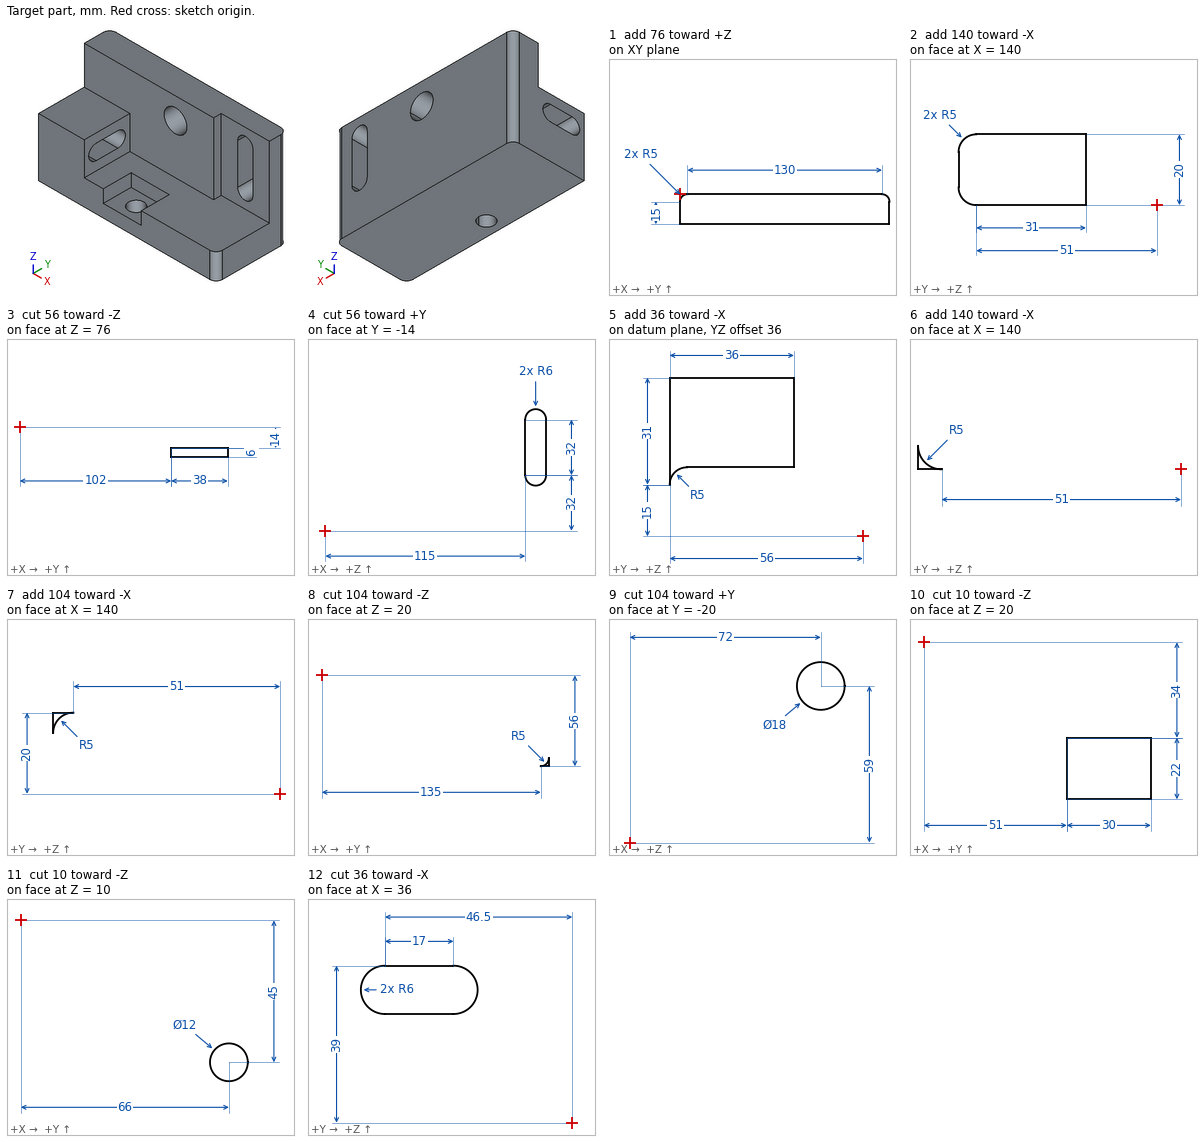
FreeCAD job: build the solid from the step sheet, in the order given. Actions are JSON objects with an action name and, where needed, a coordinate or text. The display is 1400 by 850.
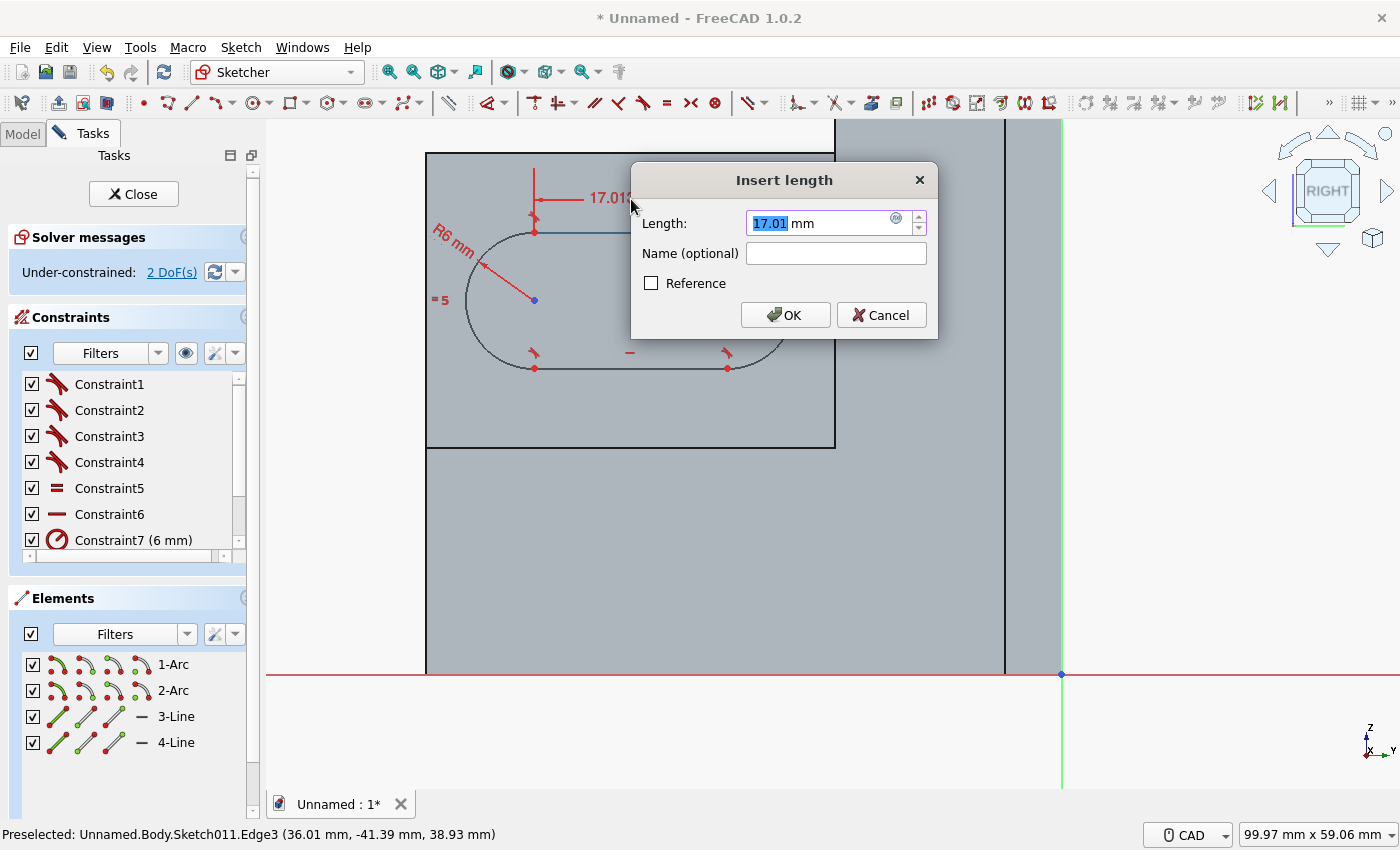
{"action": "type", "text": "17"}
{"action": "key", "text": "Return"}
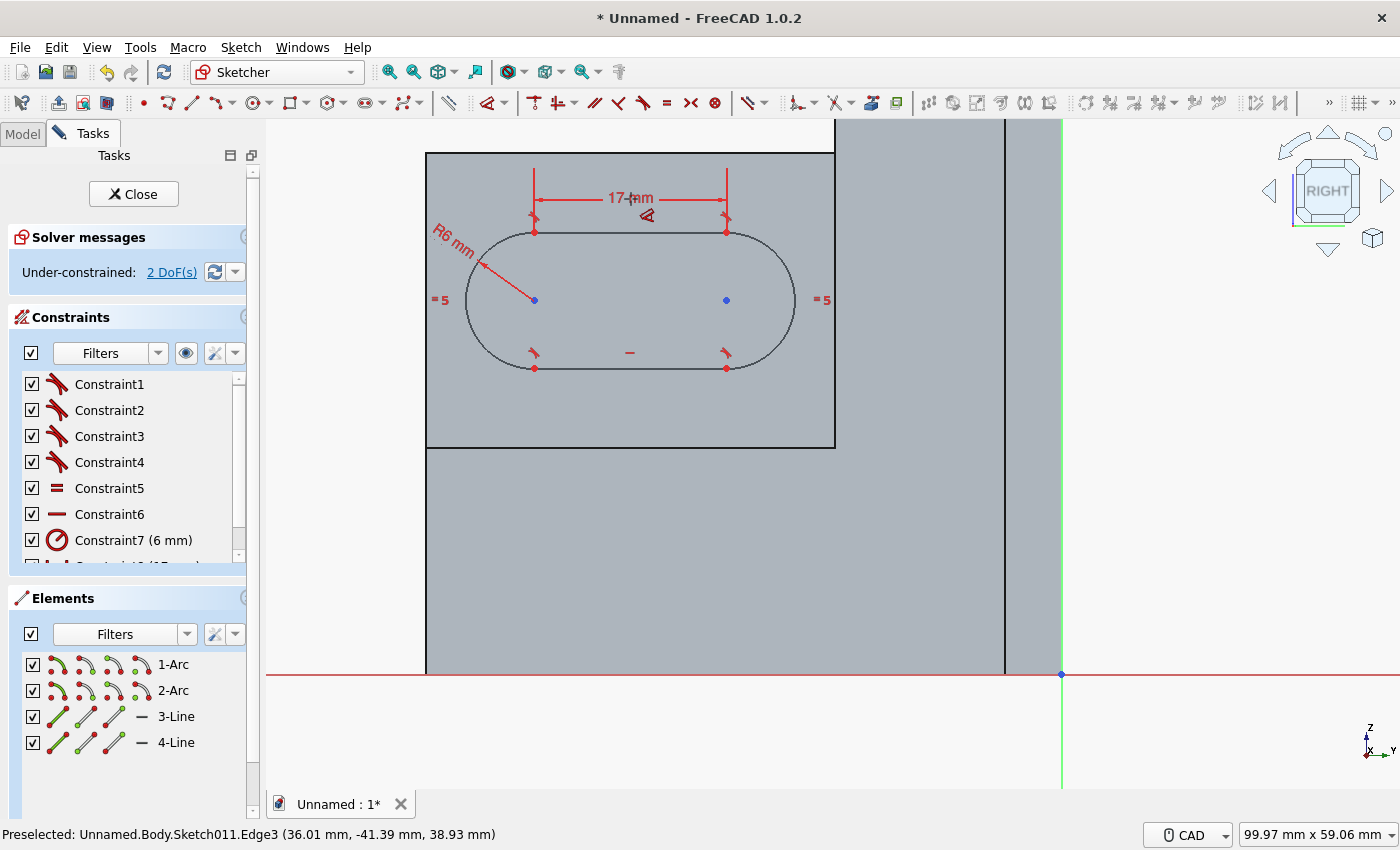
{"action": "left_click", "coordinate": [534, 233]}
{"action": "left_click", "coordinate": [1096, 454]}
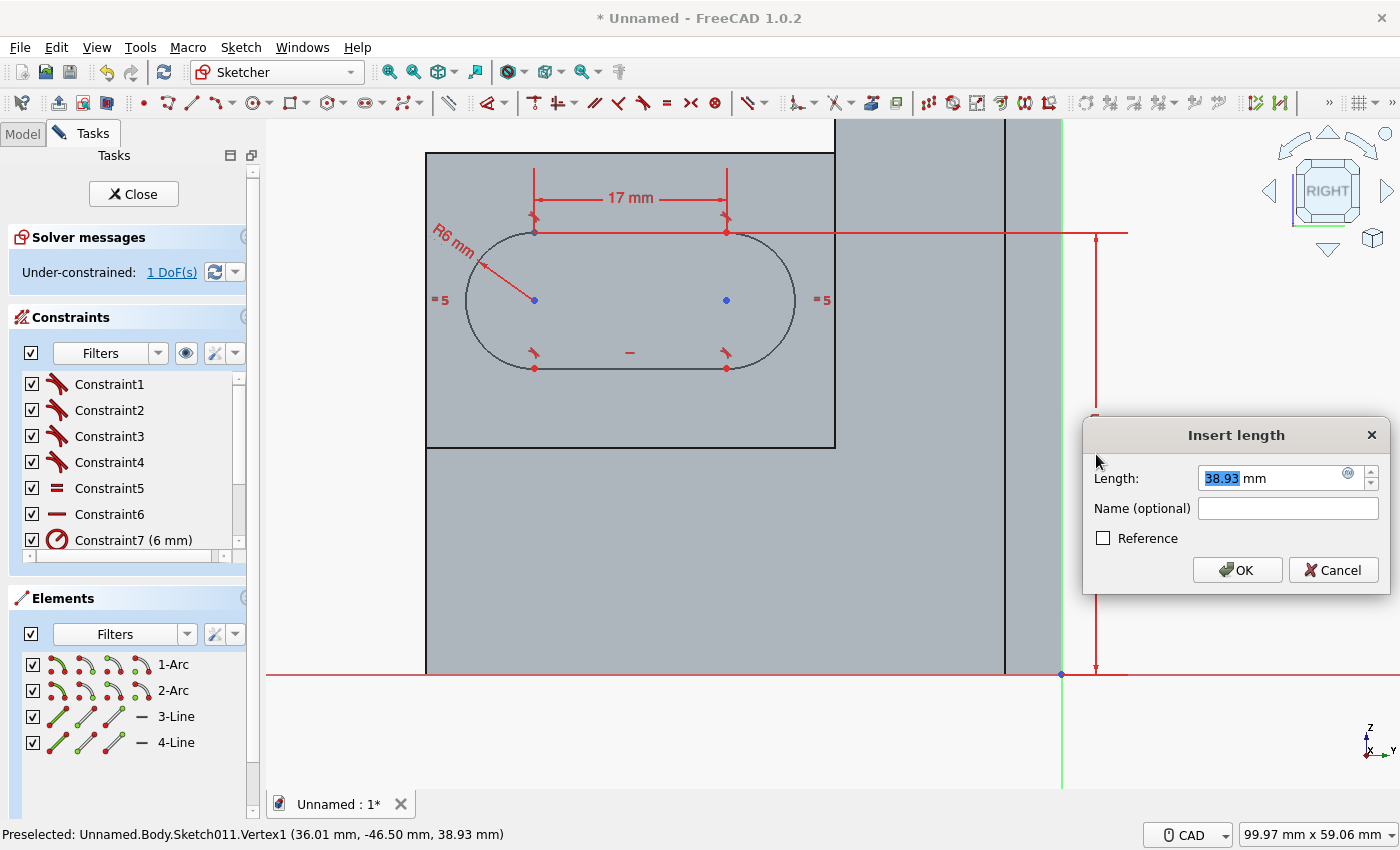
{"action": "type", "text": "39"}
{"action": "key", "text": "Return"}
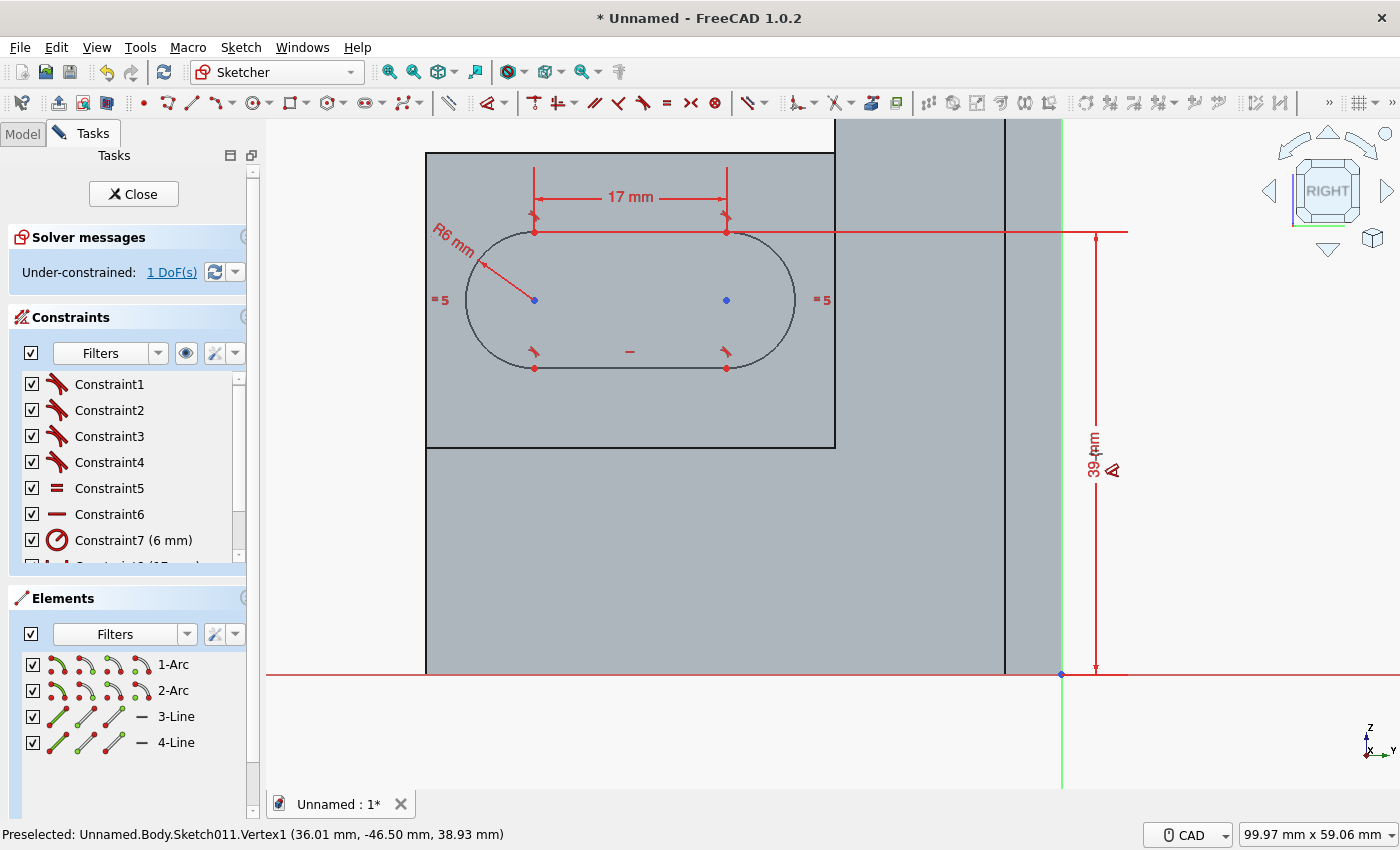
{"action": "left_click", "coordinate": [534, 232]}
{"action": "left_click", "coordinate": [798, 709]}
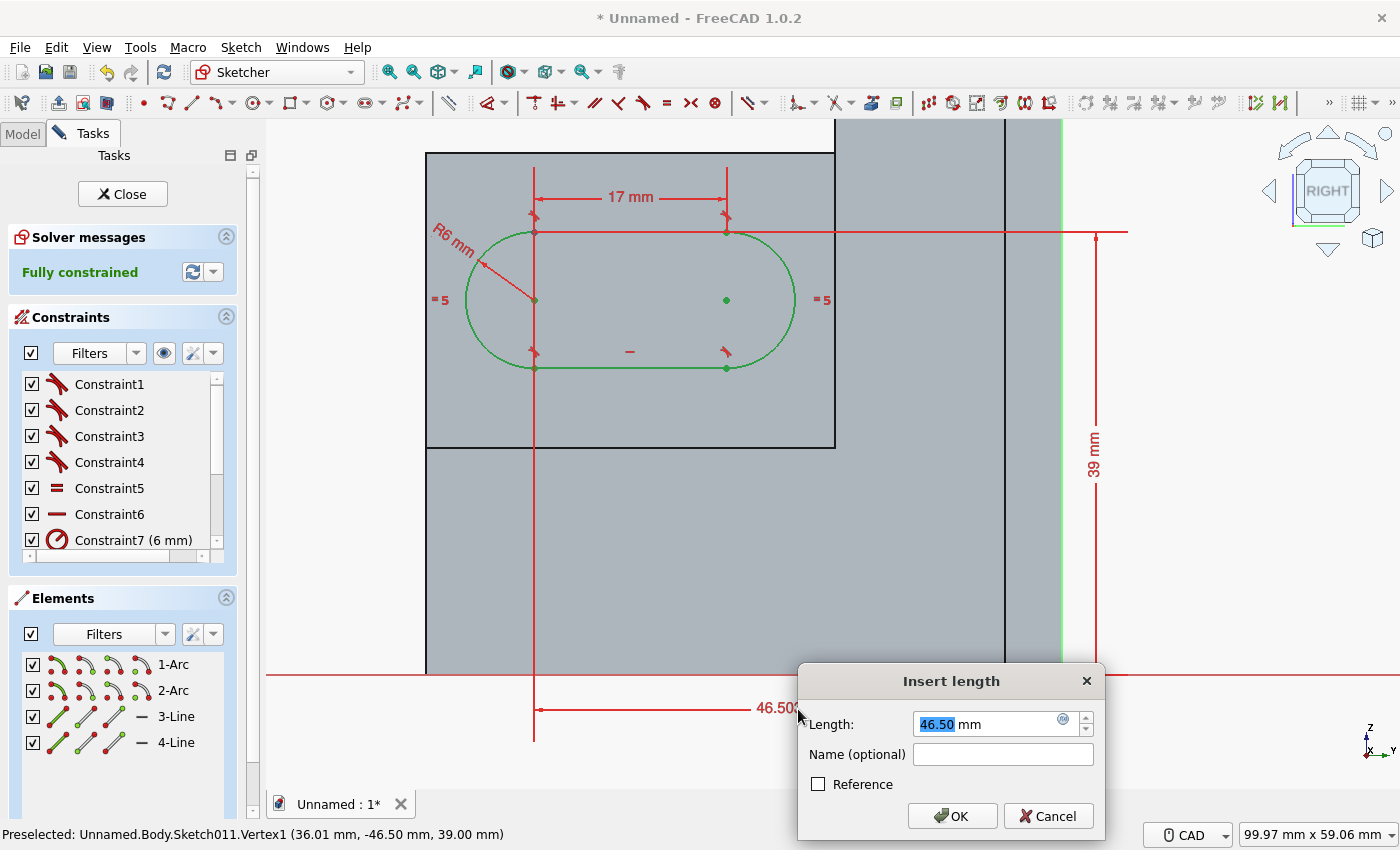
{"action": "type", "text": "46.5"}
{"action": "key", "text": "Return"}
{"action": "key", "text": "Escape"}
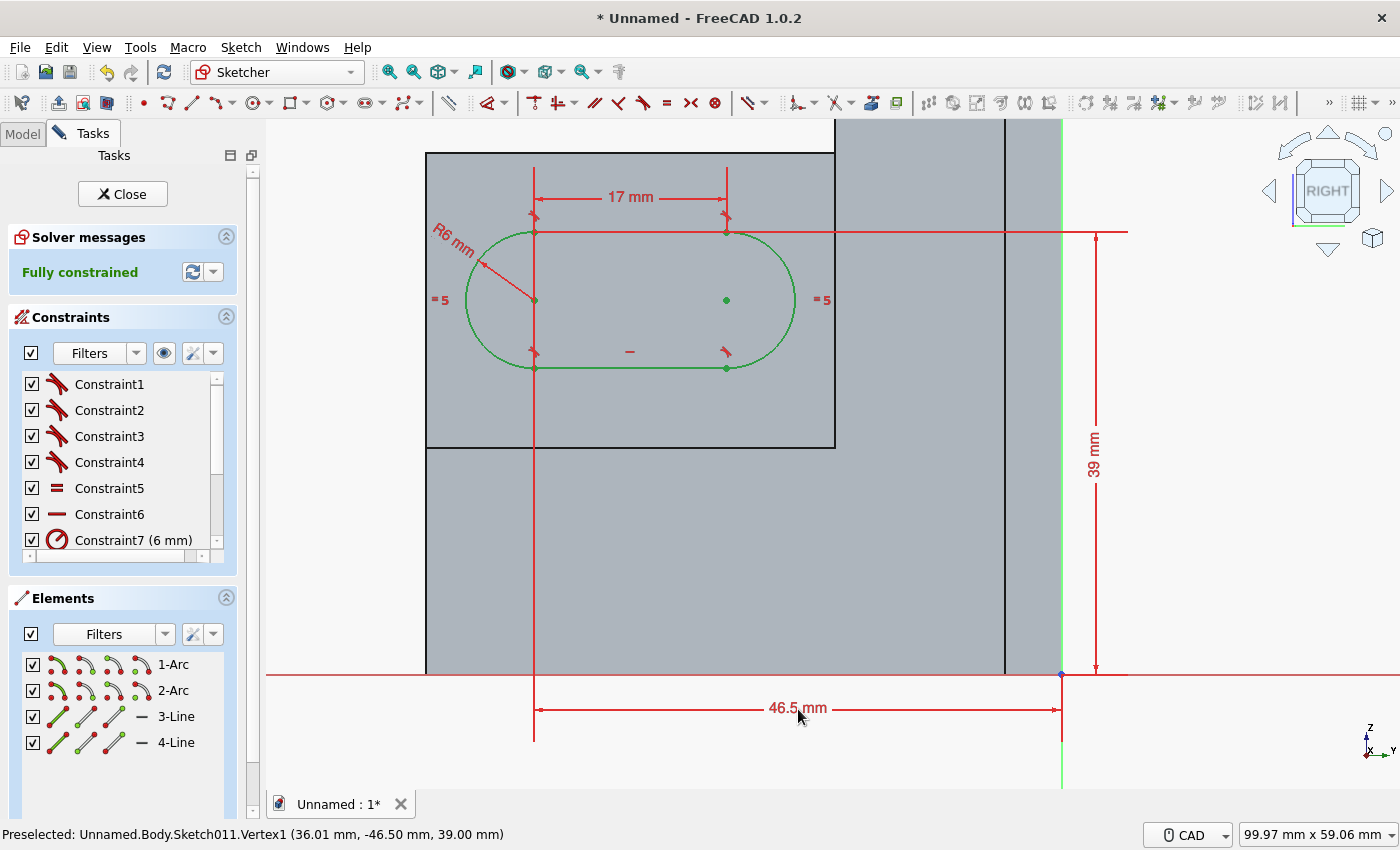
{"action": "left_click", "coordinate": [123, 194]}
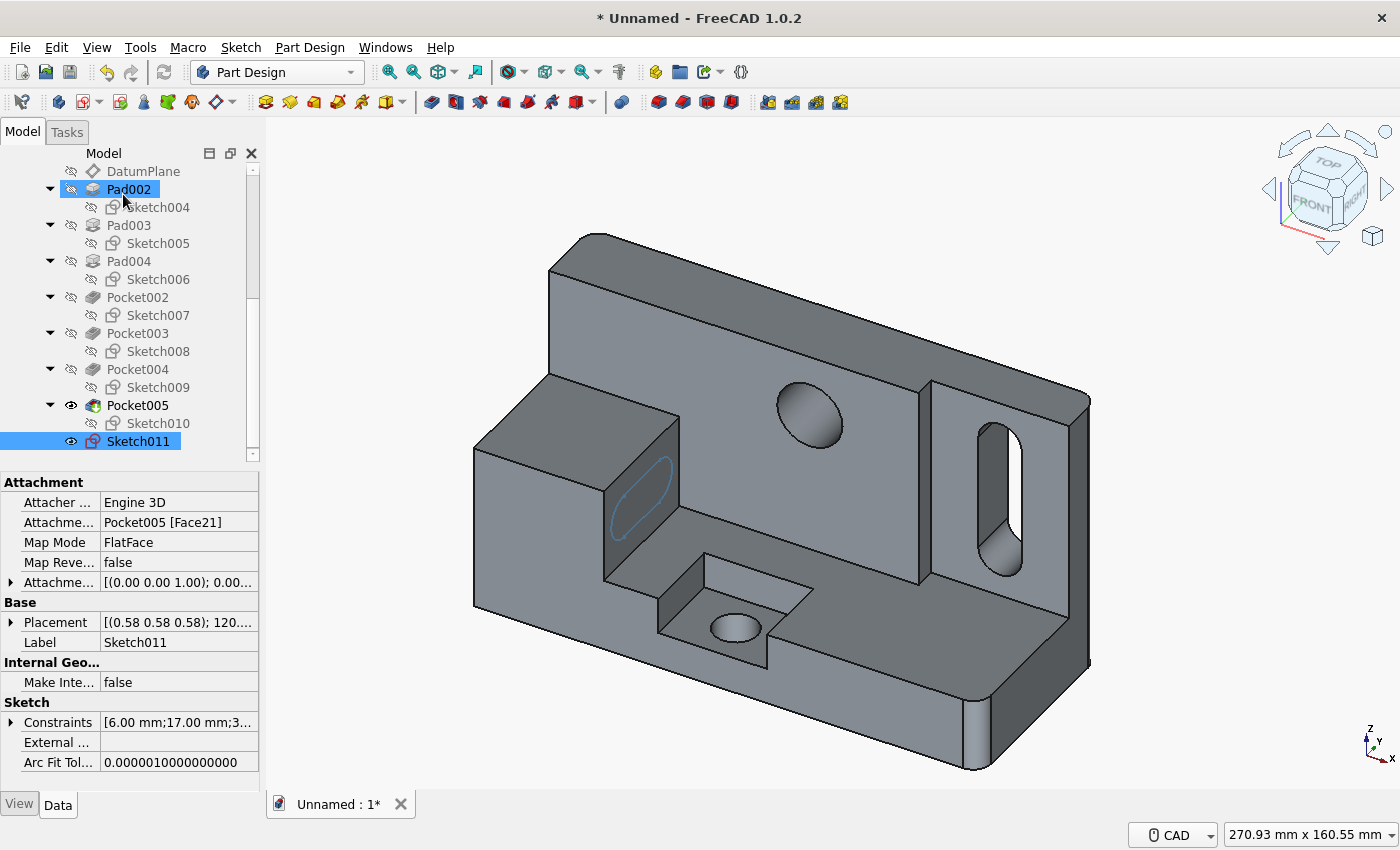
{"action": "left_click", "coordinate": [432, 102]}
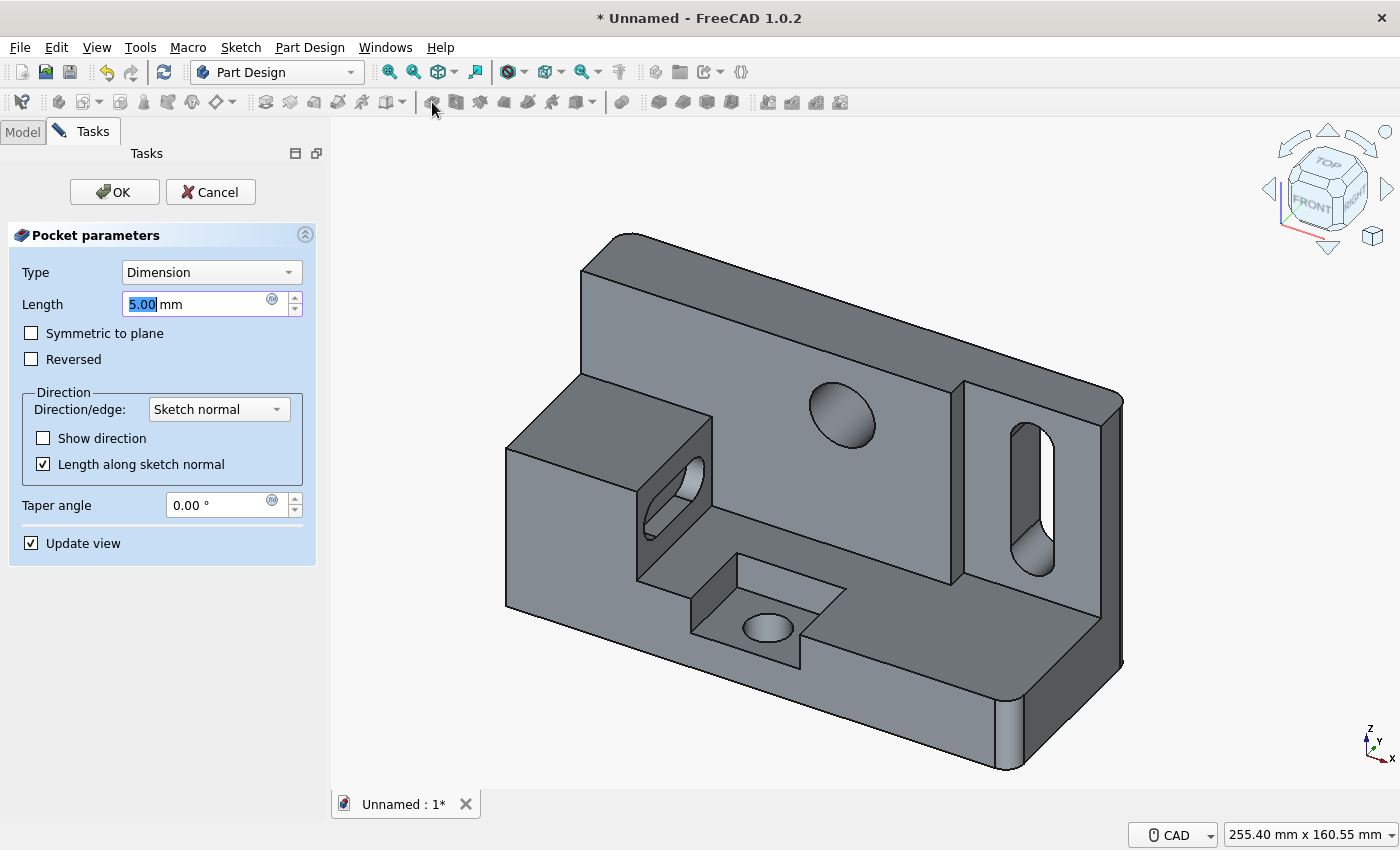
{"action": "type", "text": "36"}
{"action": "key", "text": "Tab"}